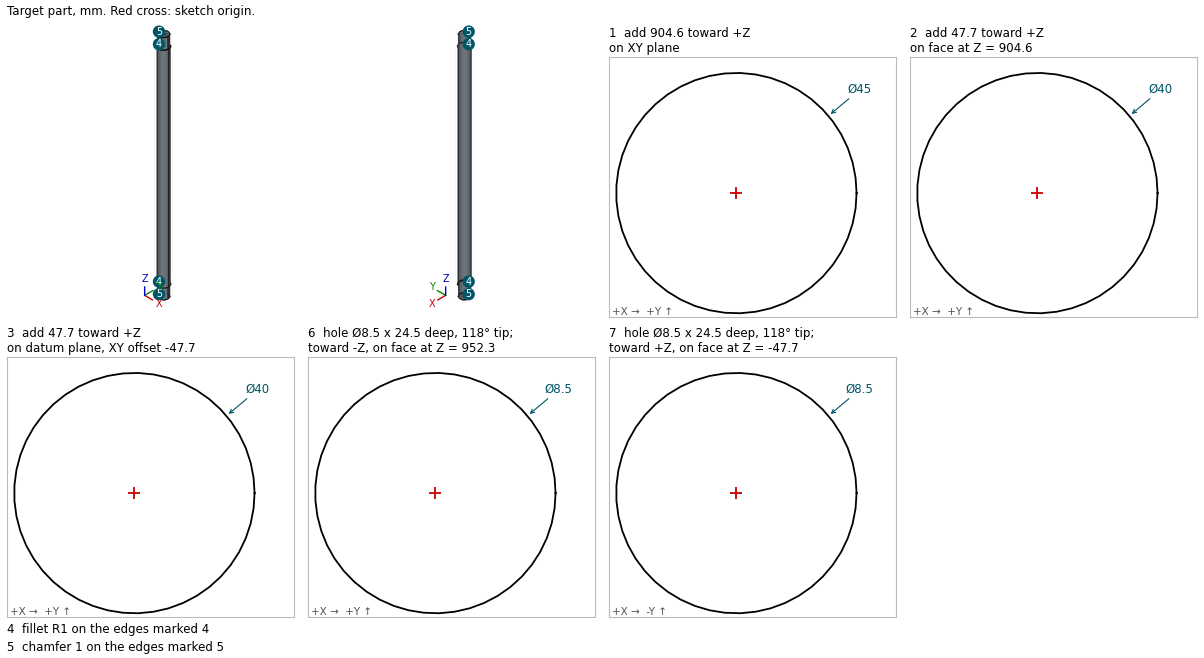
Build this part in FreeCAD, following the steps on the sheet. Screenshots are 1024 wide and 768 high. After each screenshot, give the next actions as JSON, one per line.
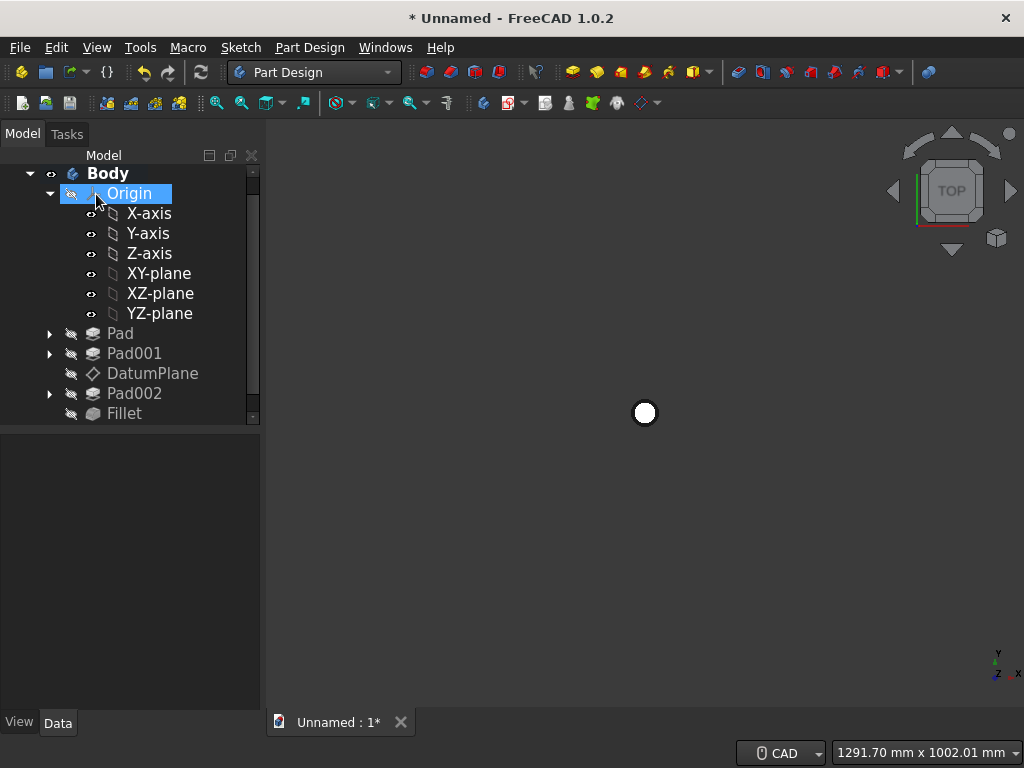
{"action": "key", "text": "v f"}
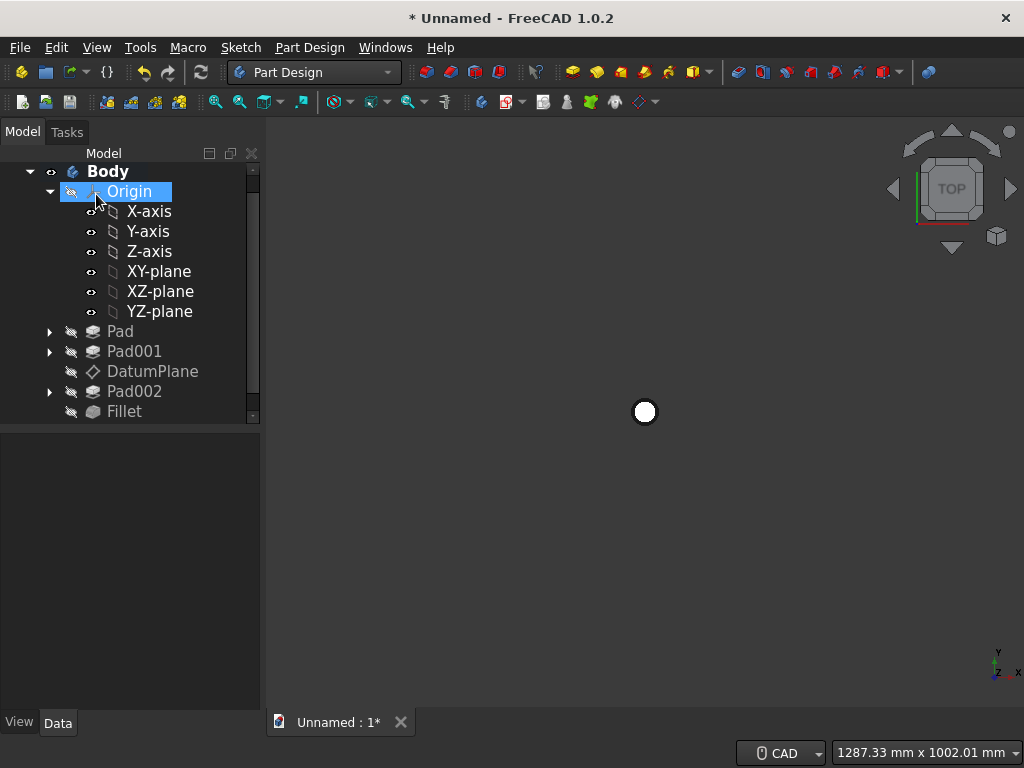
{"action": "left_click", "coordinate": [645, 411]}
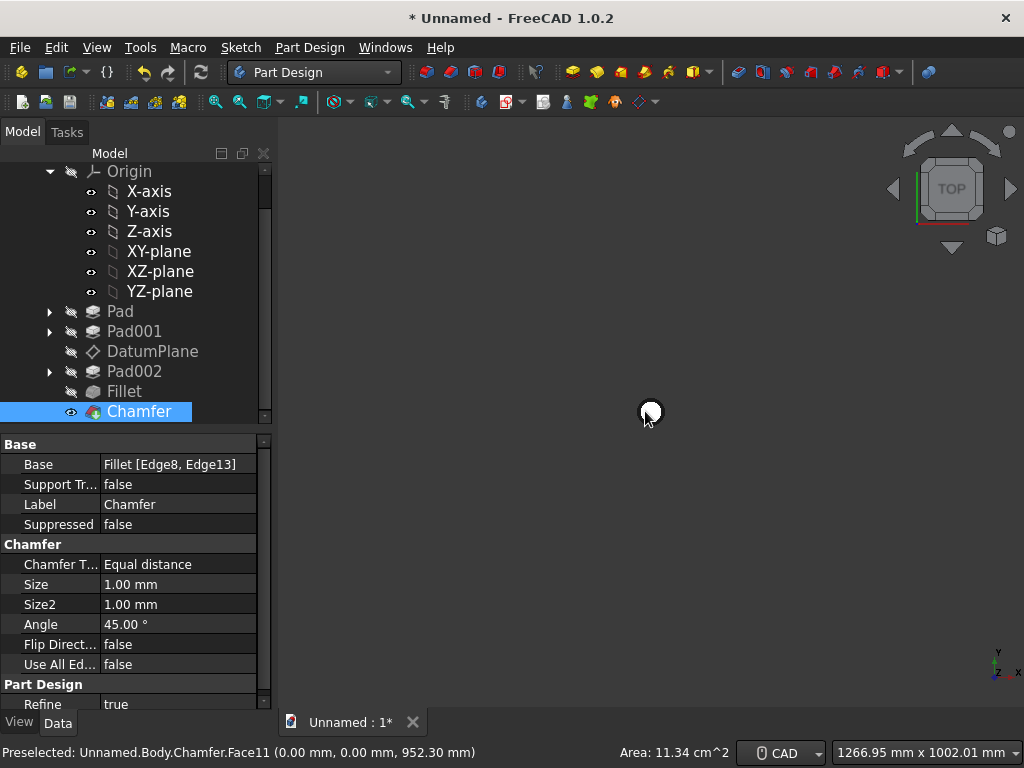
{"action": "left_click", "coordinate": [506, 102]}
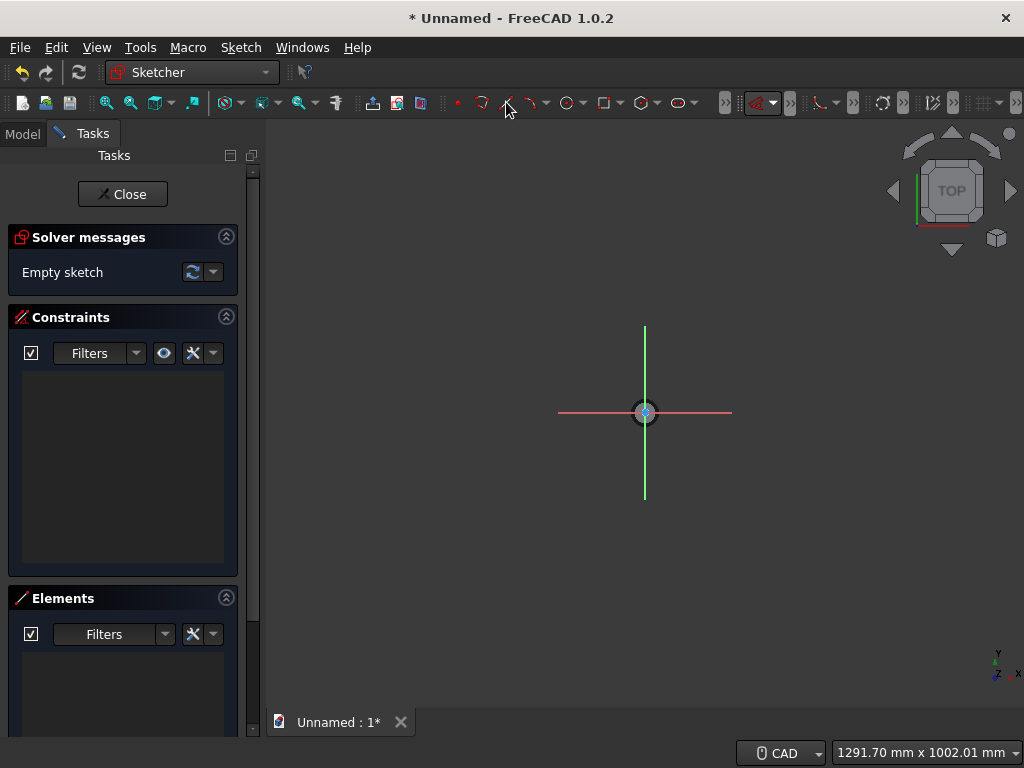
{"action": "scroll", "coordinate": [649, 413], "scroll_direction": "up", "scroll_amount": 15}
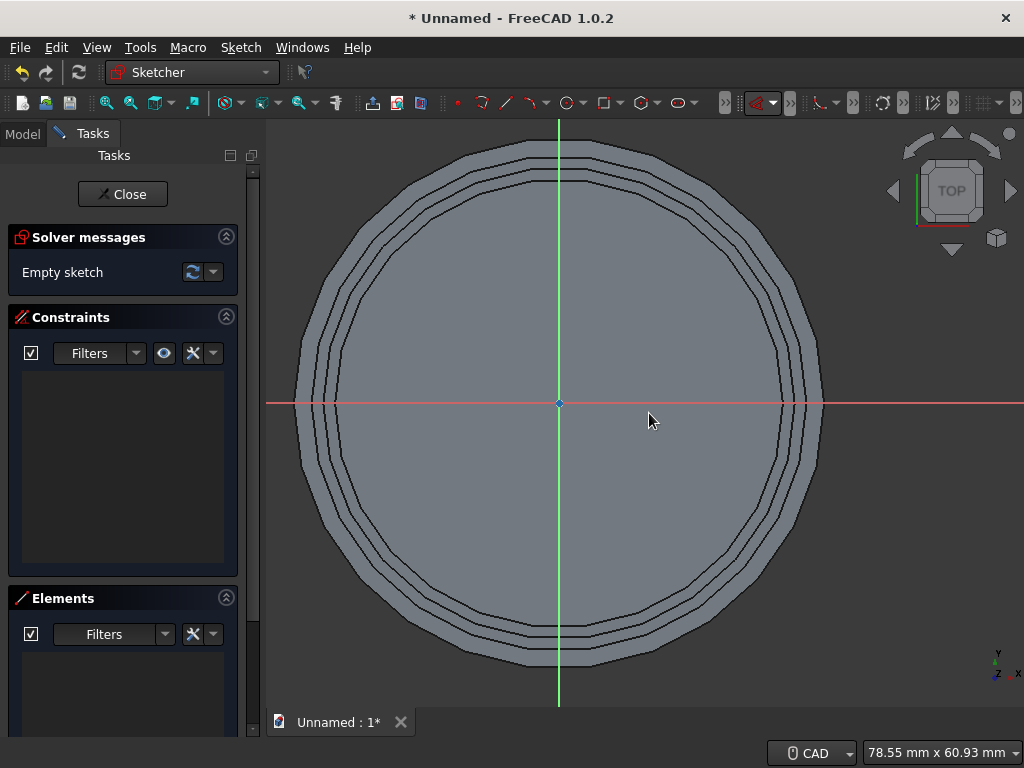
{"action": "scroll", "coordinate": [553, 400], "scroll_direction": "up", "scroll_amount": 7}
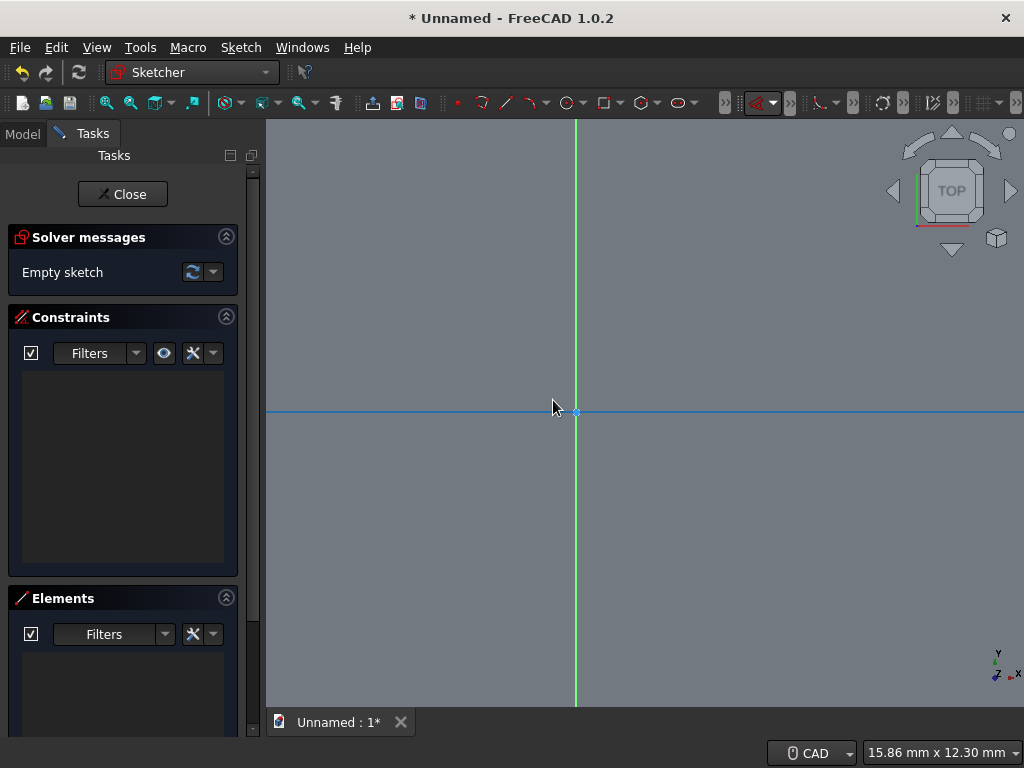
{"action": "left_click", "coordinate": [568, 104]}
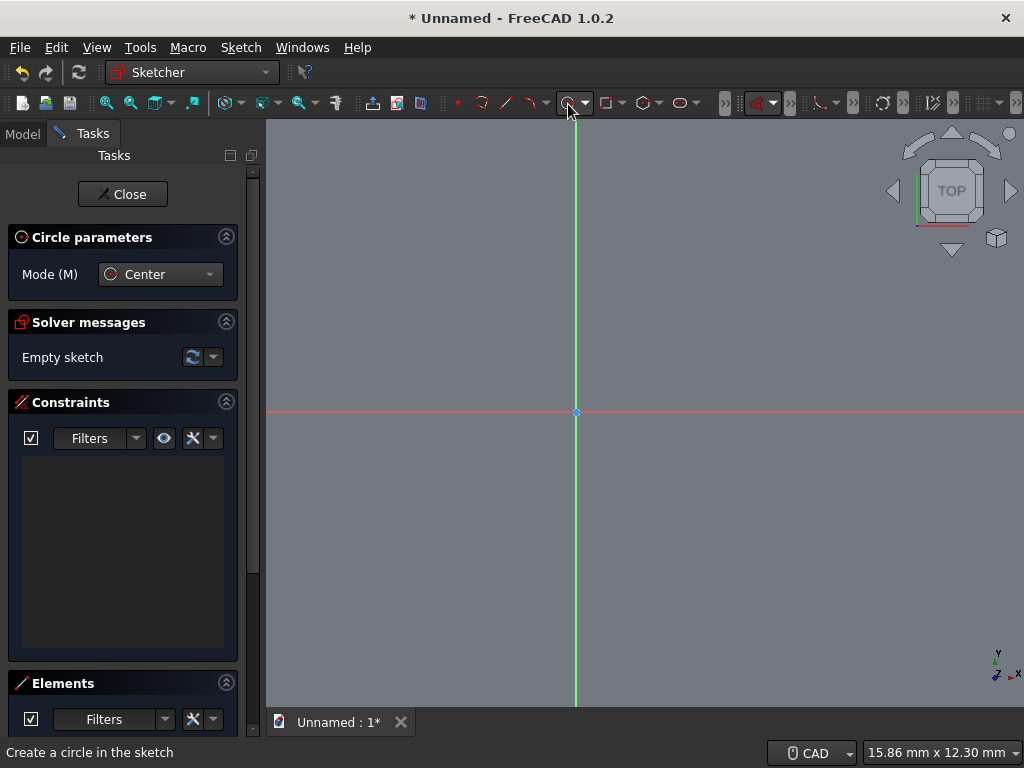
{"action": "left_click", "coordinate": [576, 412]}
{"action": "mouse_move", "coordinate": [720, 269]}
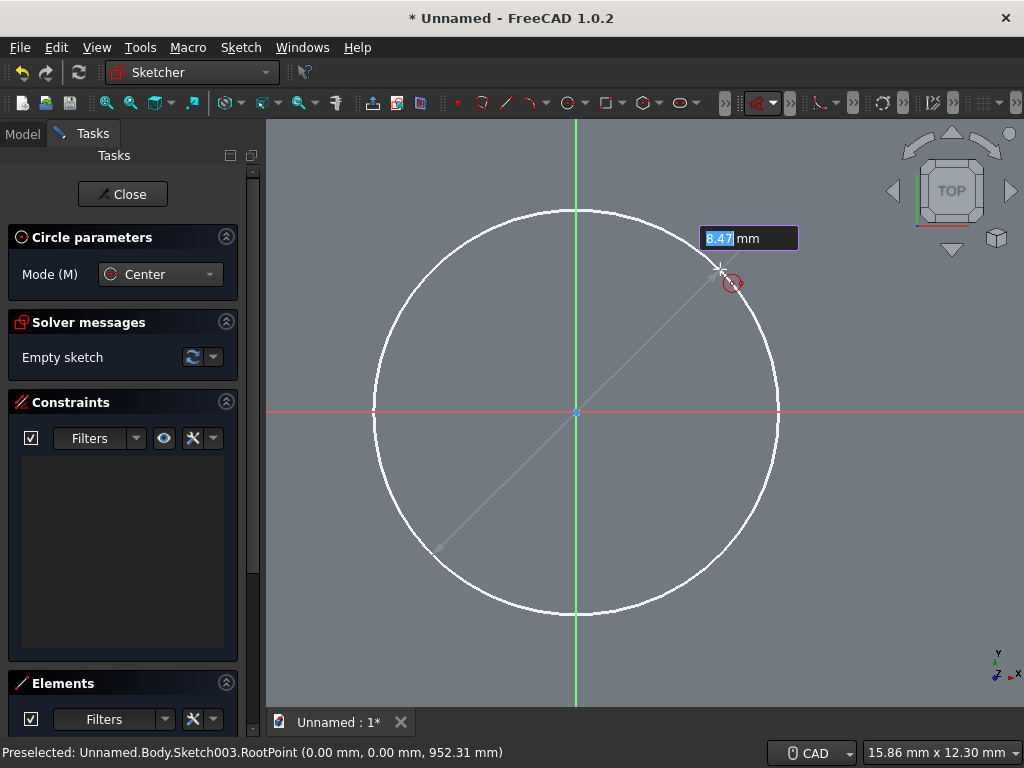
{"action": "type", "text": "8.5"}
{"action": "key", "text": "Return"}
{"action": "key", "text": "Escape"}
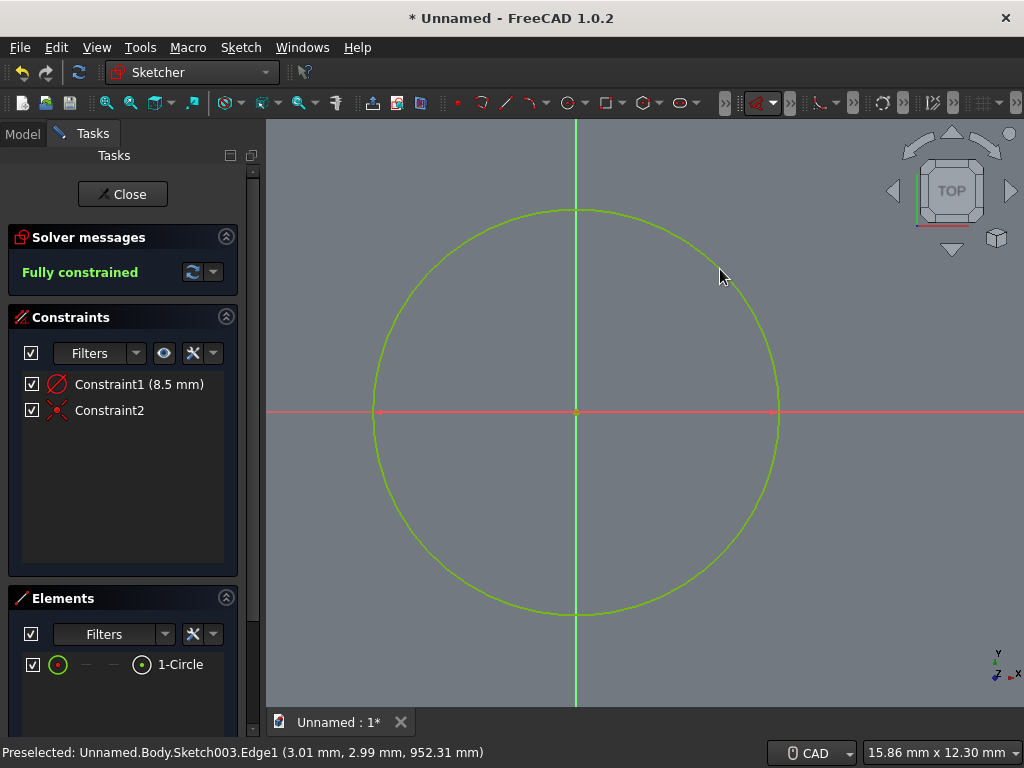
{"action": "left_click", "coordinate": [123, 194]}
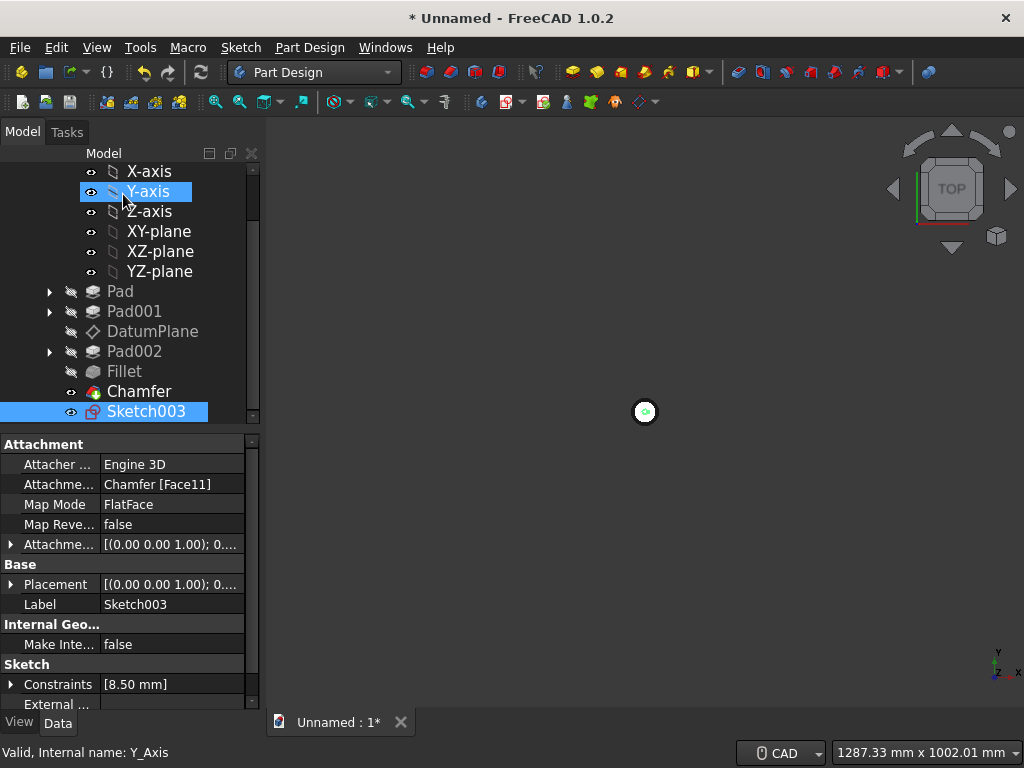
{"action": "left_click", "coordinate": [764, 72]}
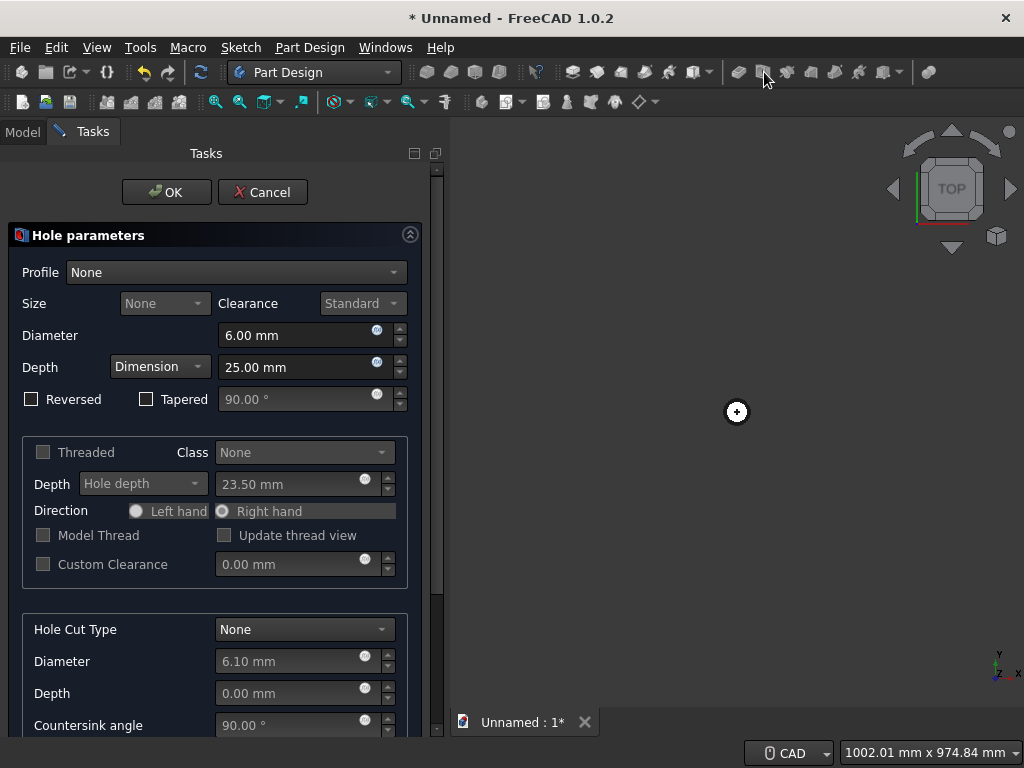
{"action": "triple_click", "coordinate": [305, 335]}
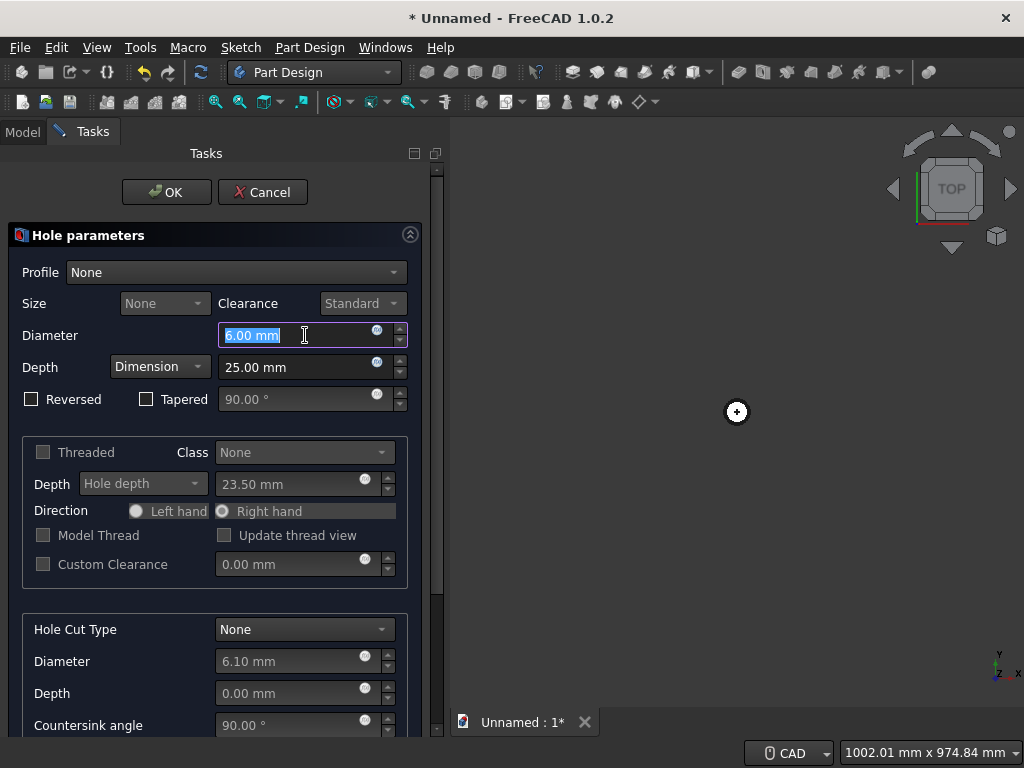
{"action": "type", "text": "8.5"}
{"action": "key", "text": "Tab"}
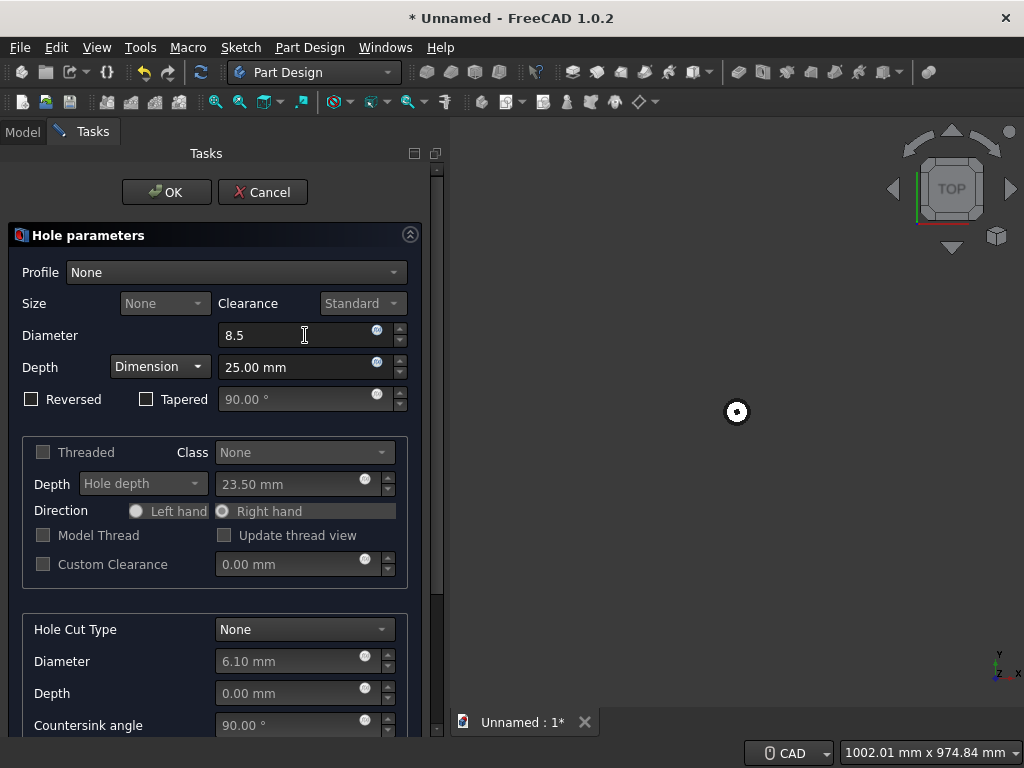
{"action": "triple_click", "coordinate": [305, 367]}